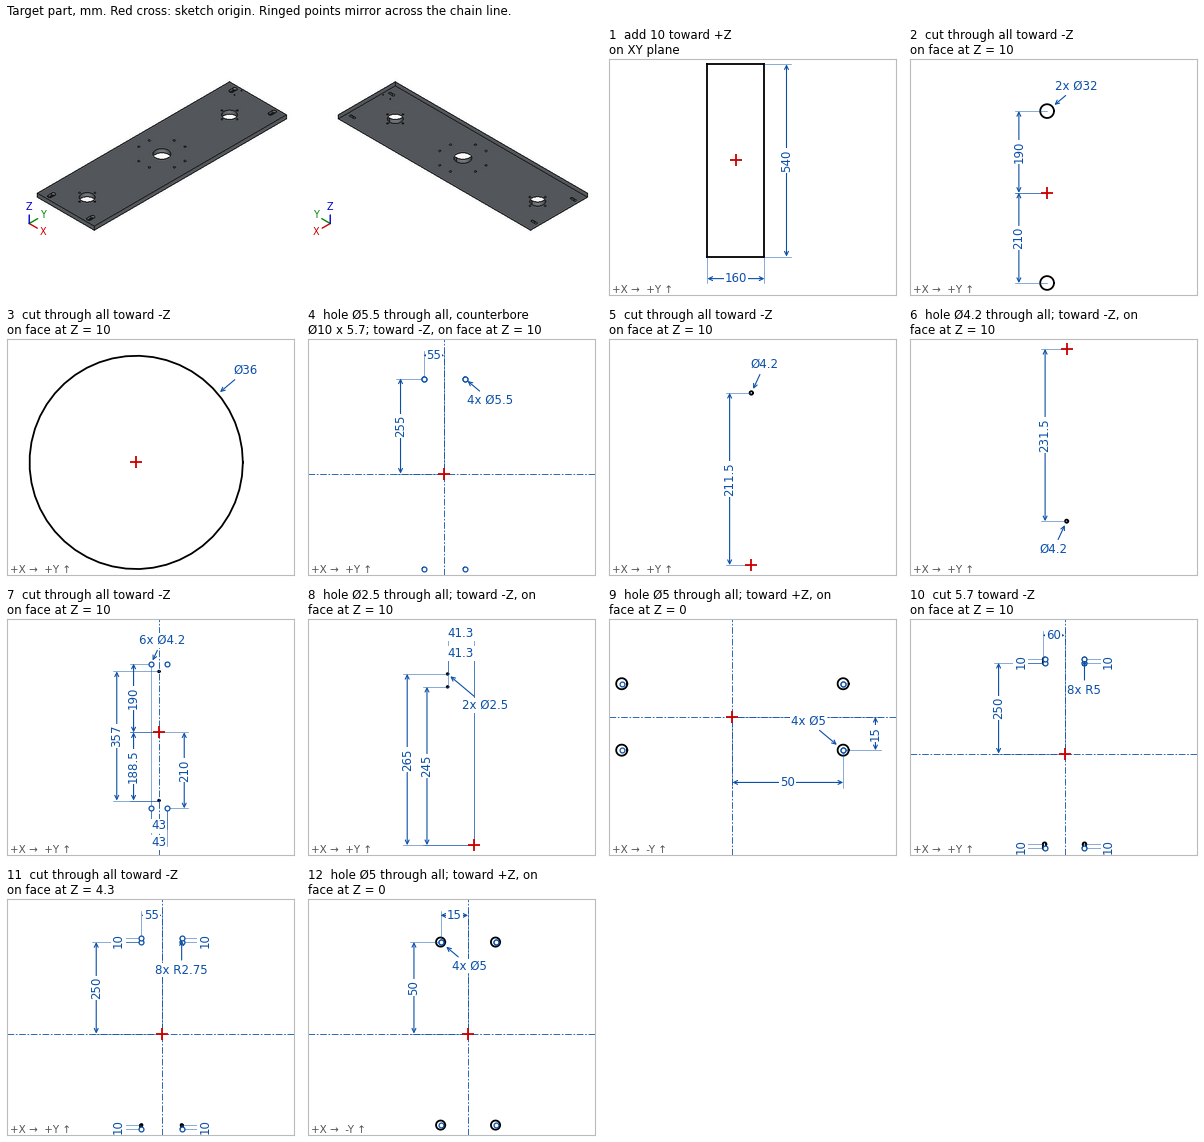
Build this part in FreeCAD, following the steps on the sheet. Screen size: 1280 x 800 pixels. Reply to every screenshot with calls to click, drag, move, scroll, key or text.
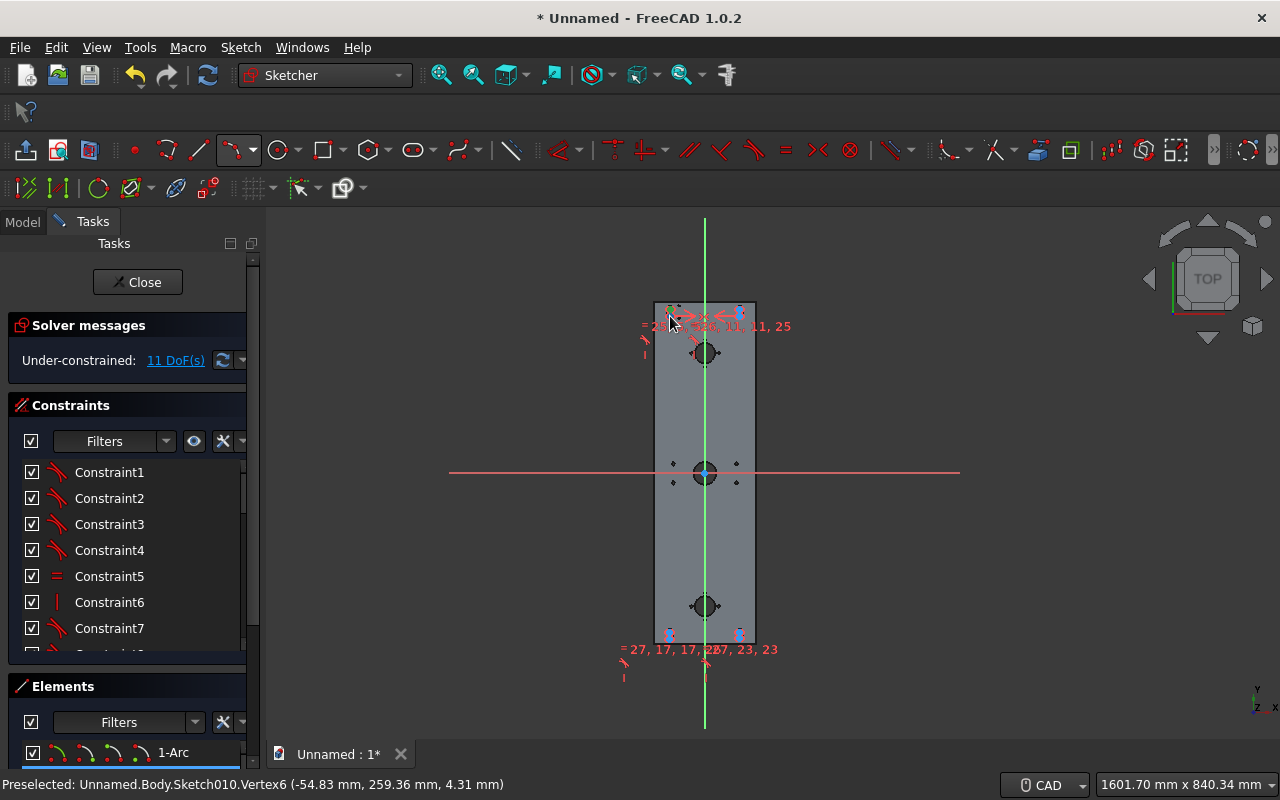
scroll(670, 639, up, 9)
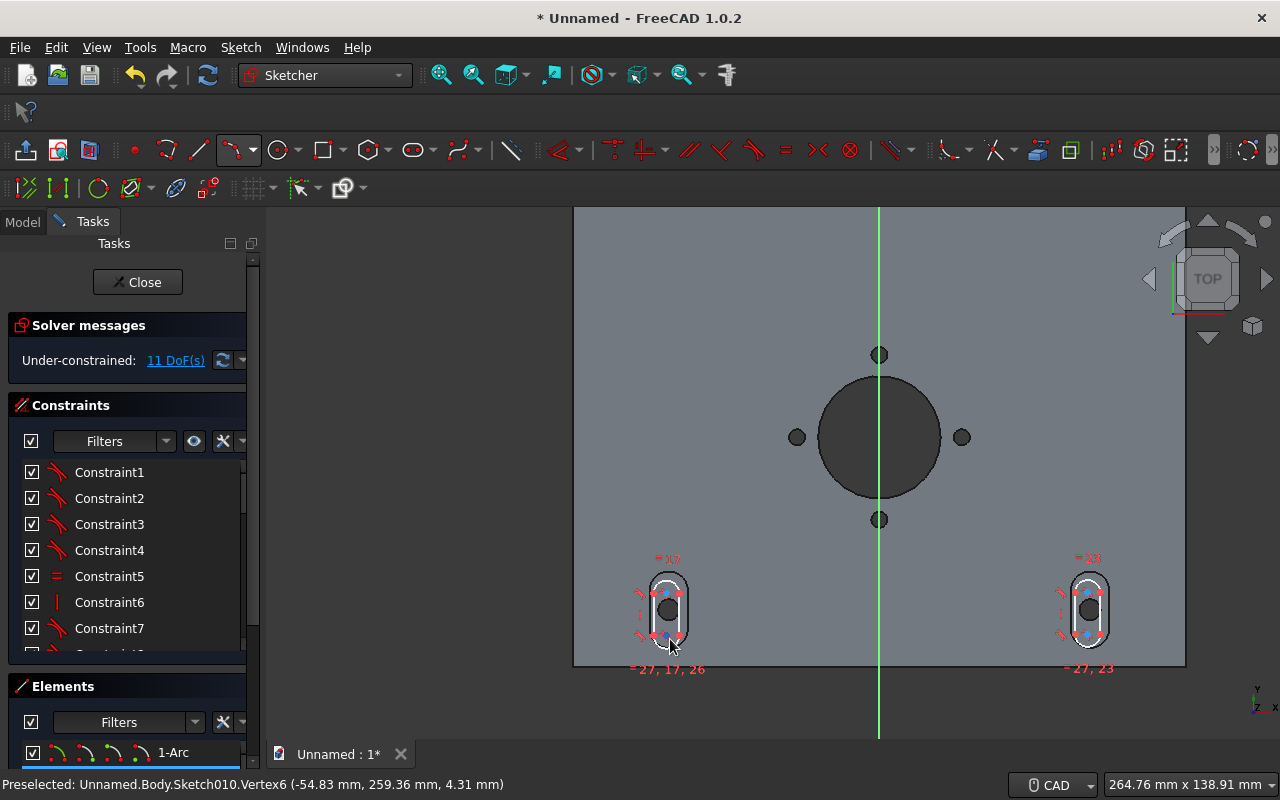
click(666, 636)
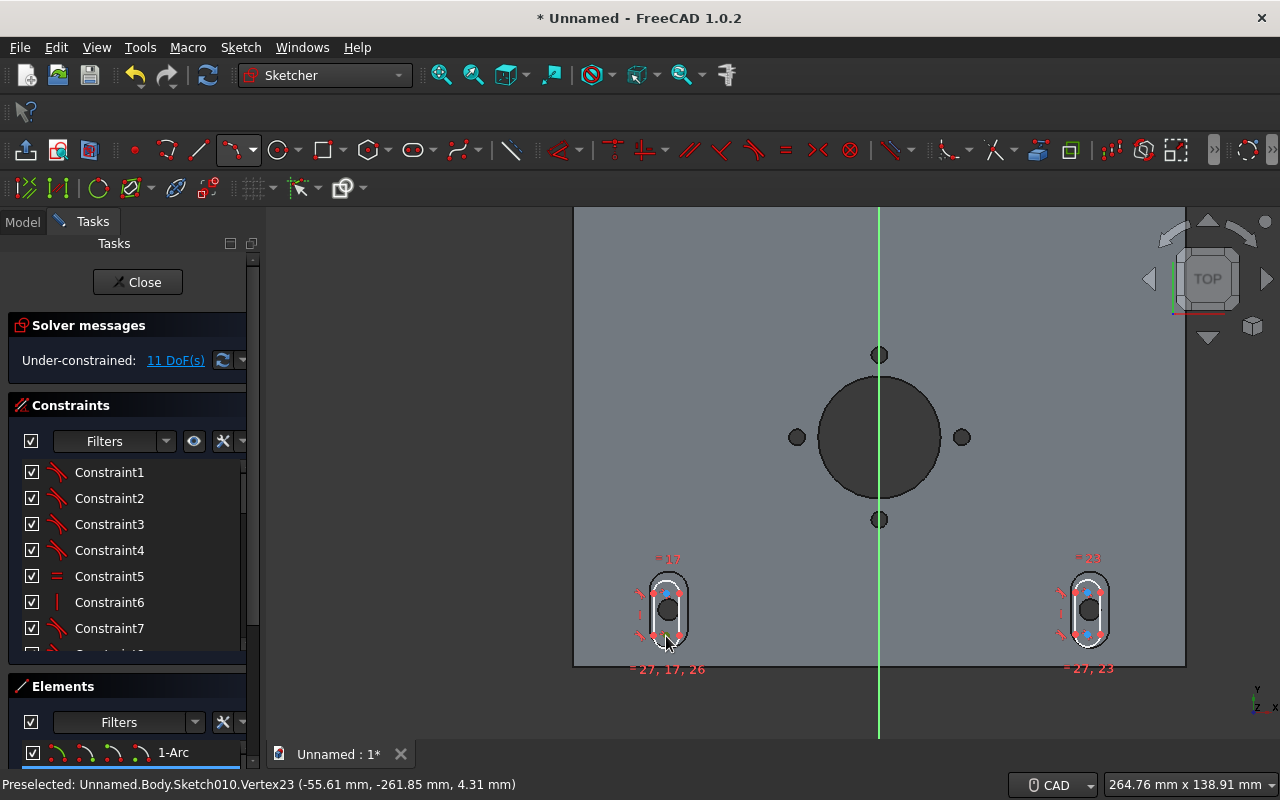
scroll(670, 639, down, 9)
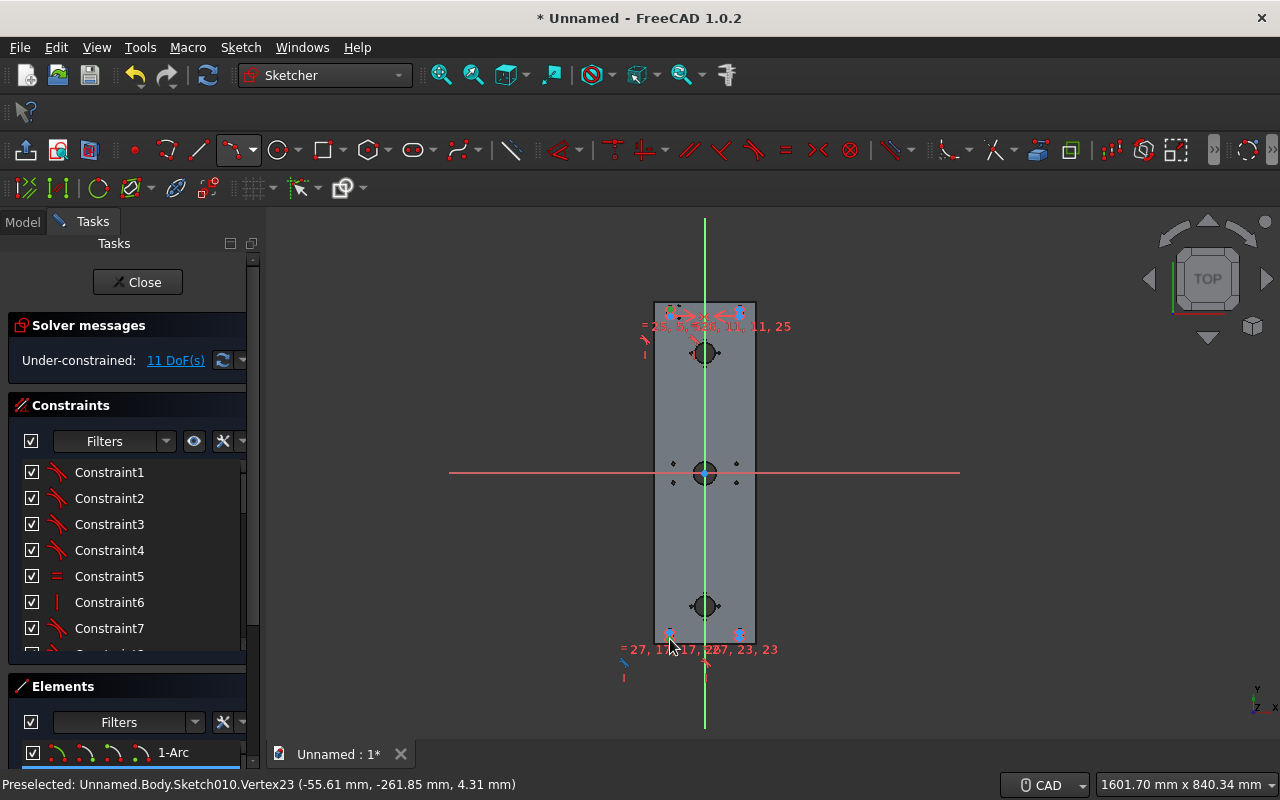
click(470, 473)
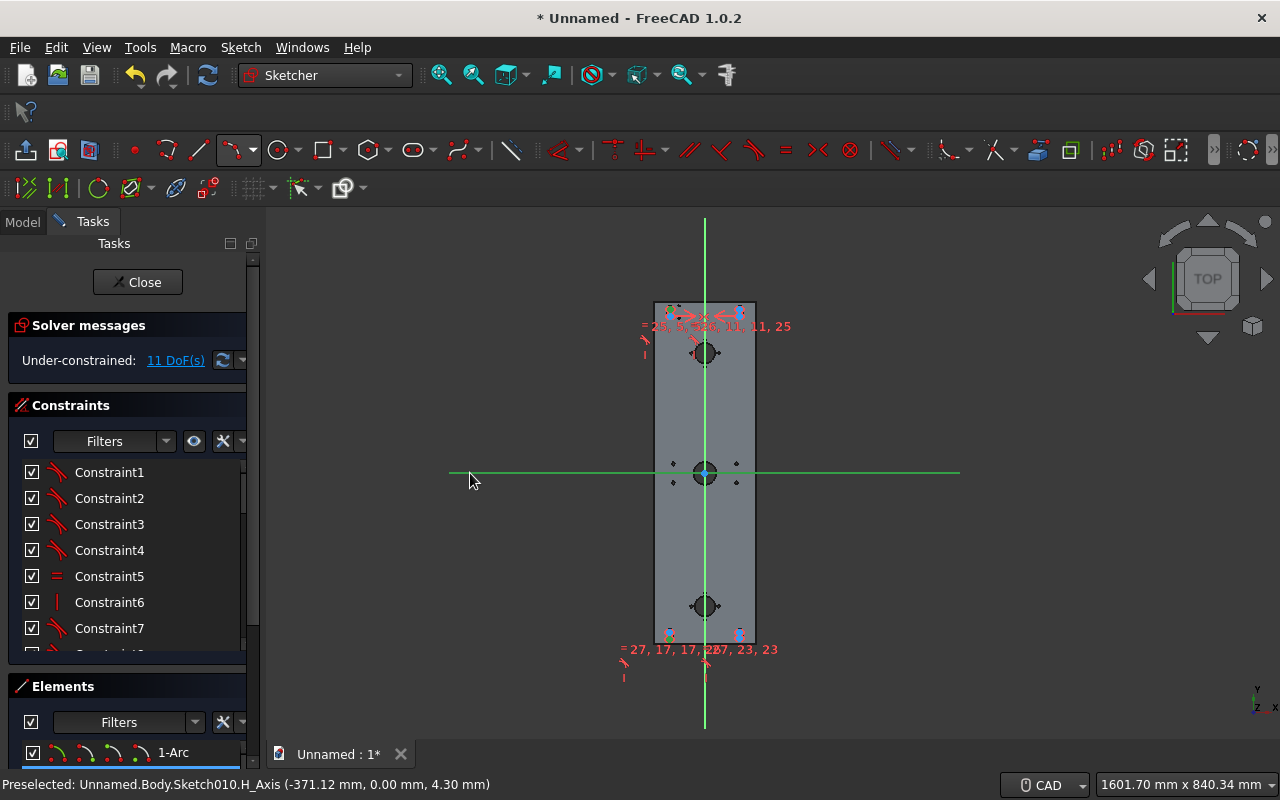
click(818, 150)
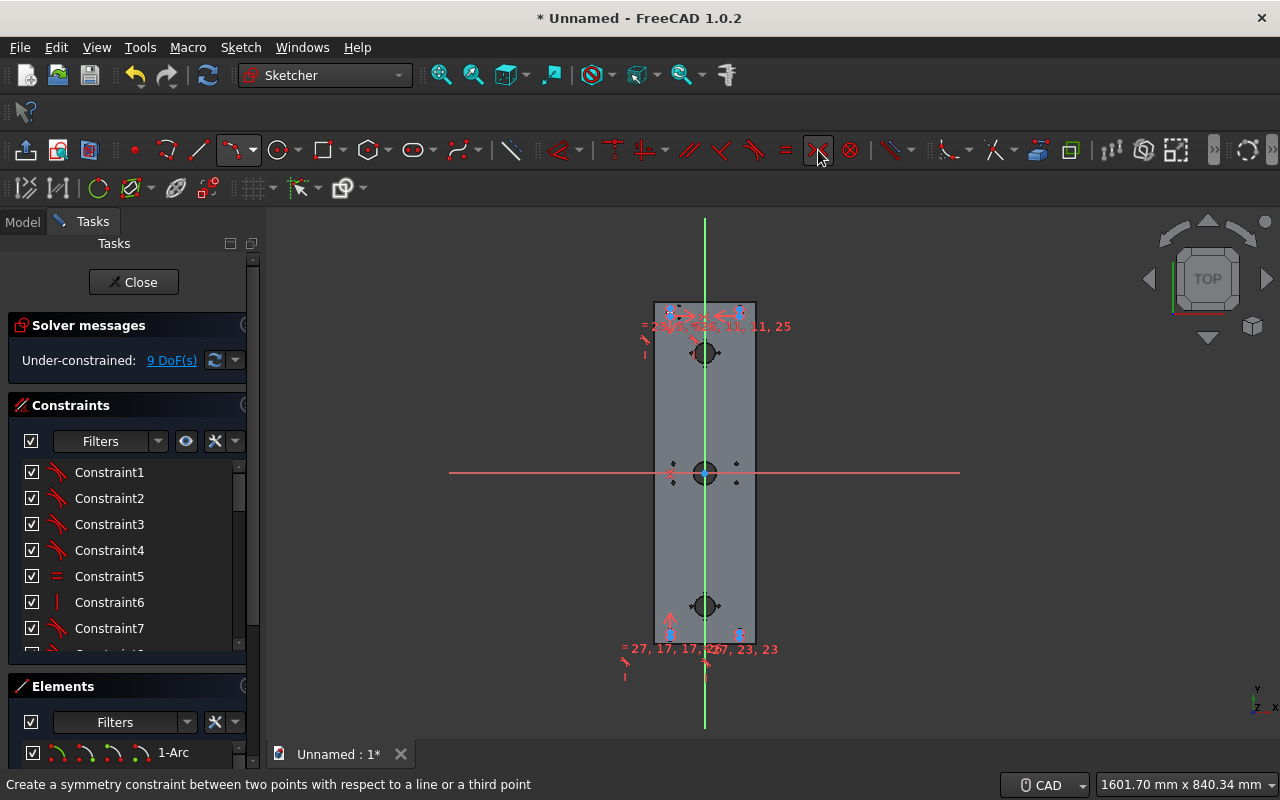
scroll(740, 309, up, 9)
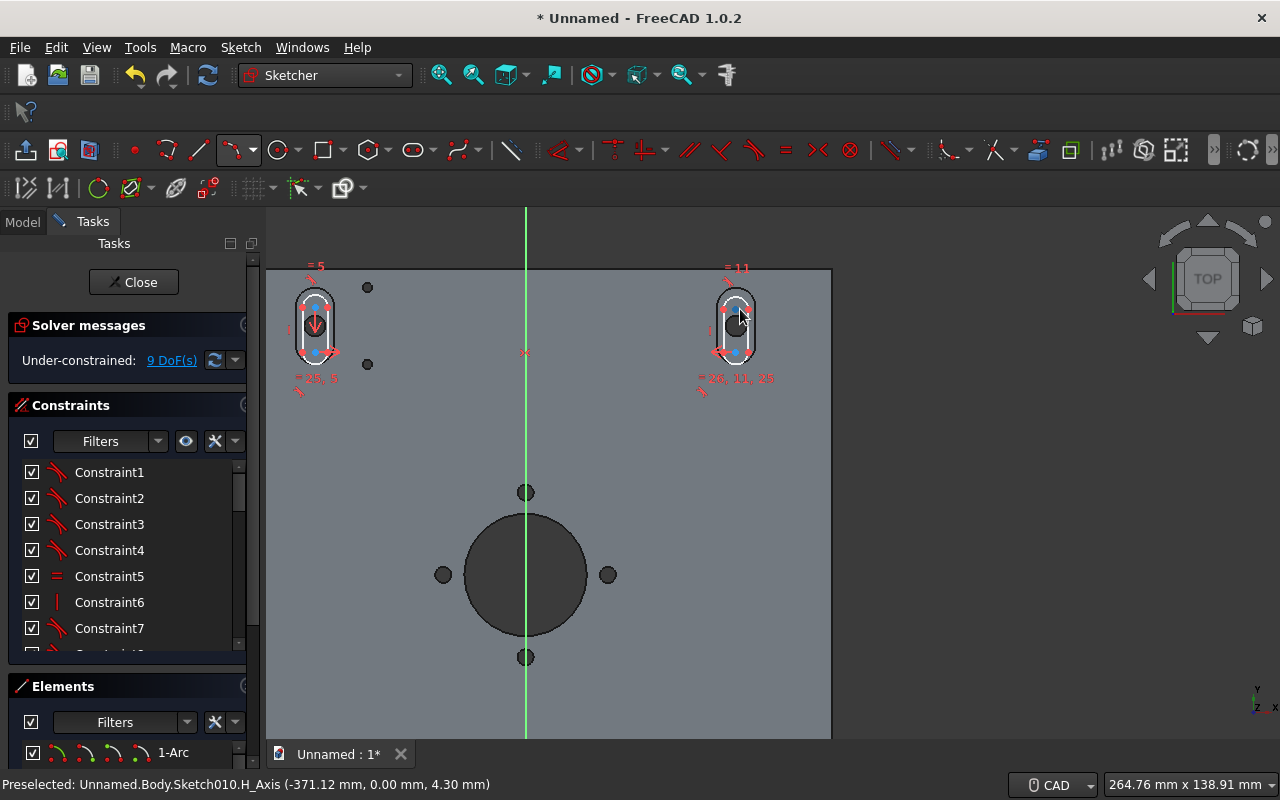
click(736, 309)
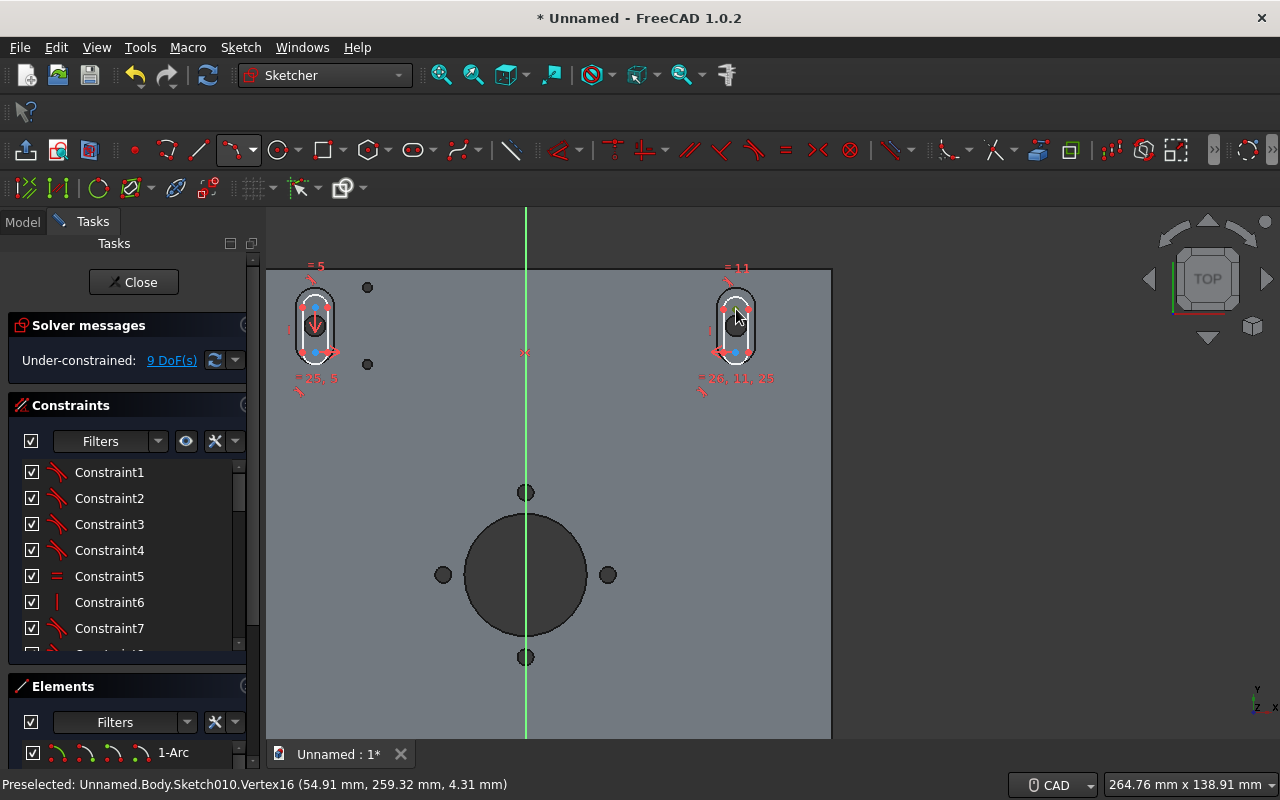
scroll(740, 309, down, 9)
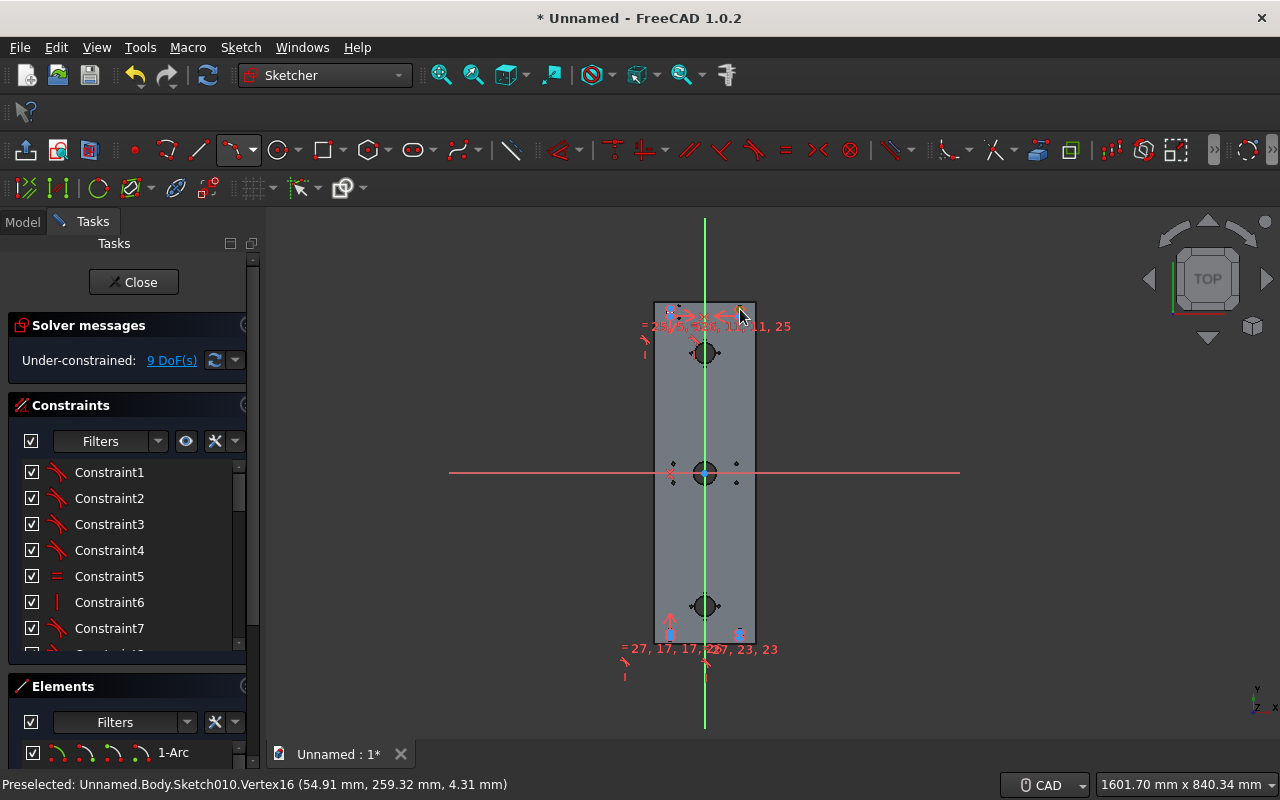
scroll(739, 639, up, 9)